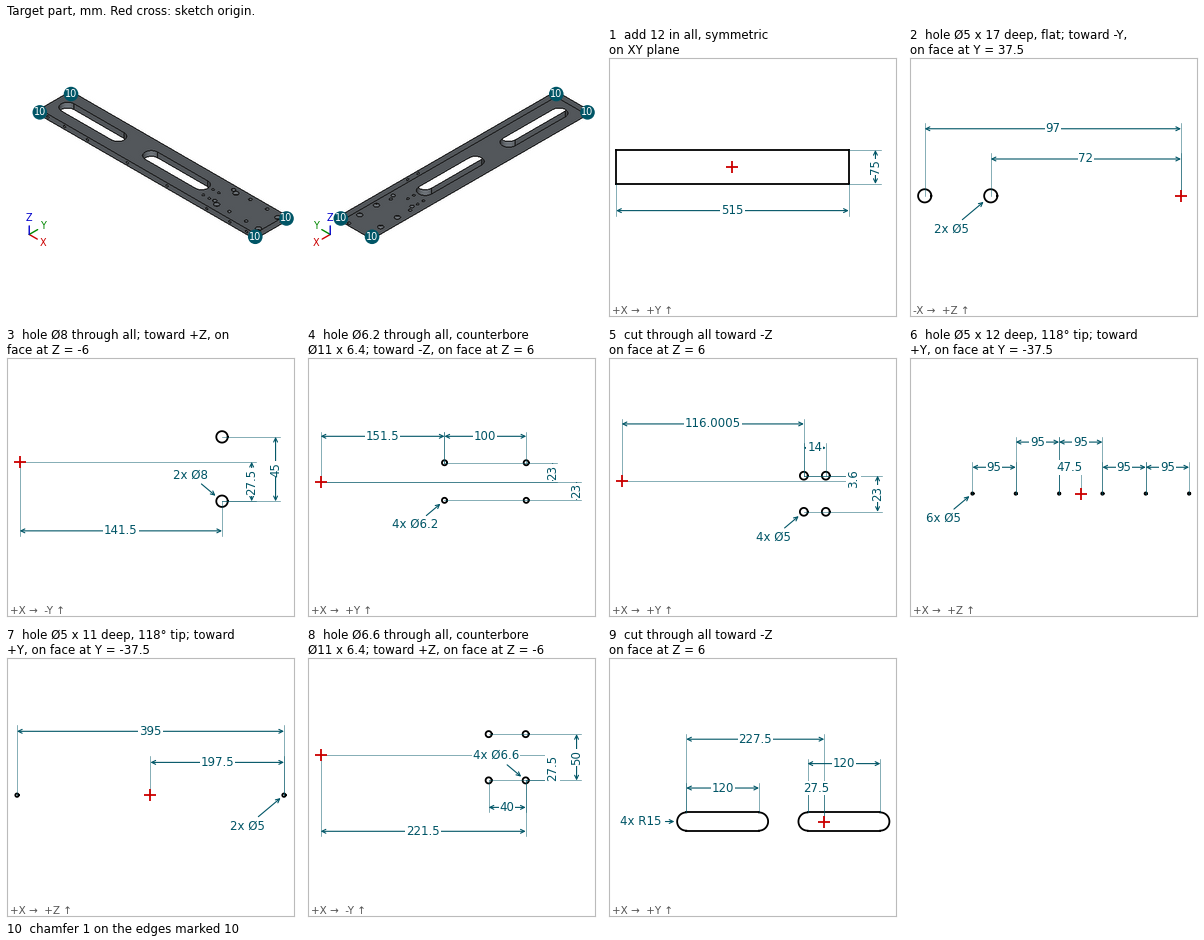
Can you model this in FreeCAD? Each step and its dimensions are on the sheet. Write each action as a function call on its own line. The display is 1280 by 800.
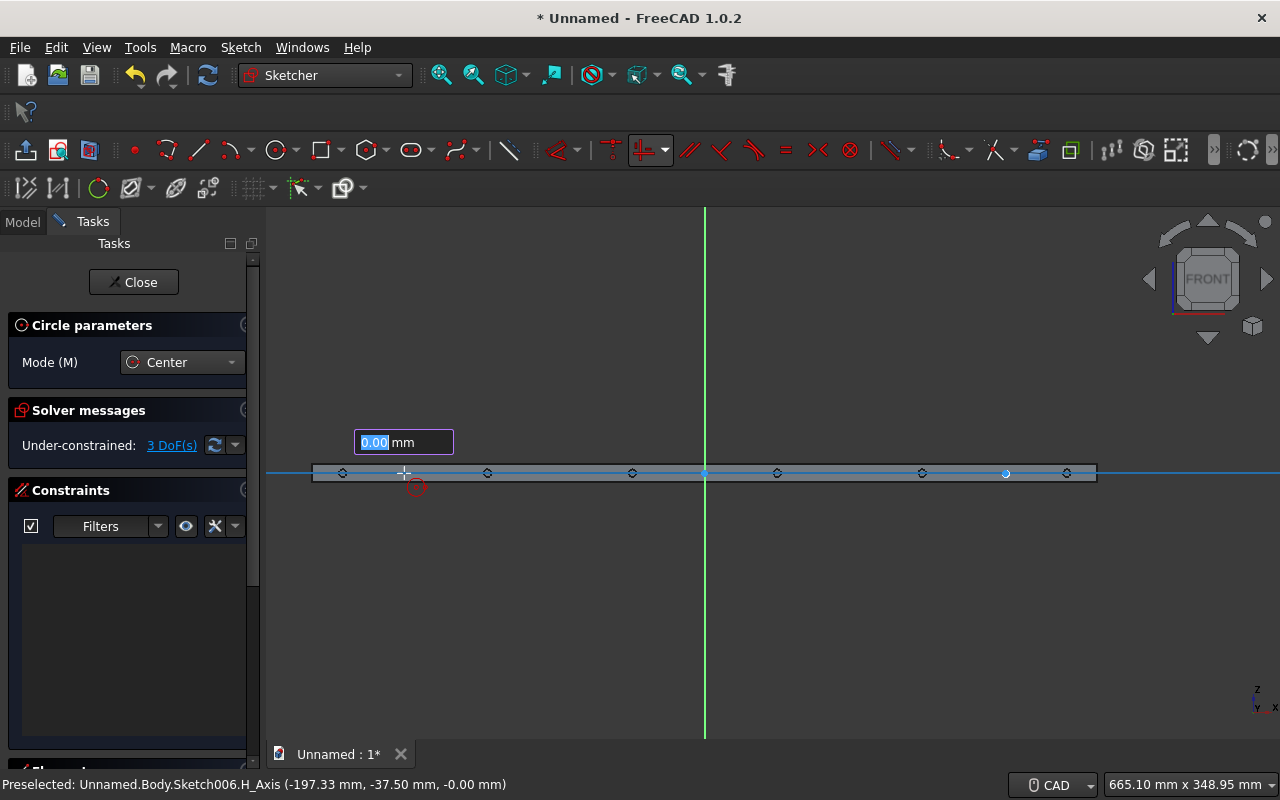
scroll(402, 477, up, 8)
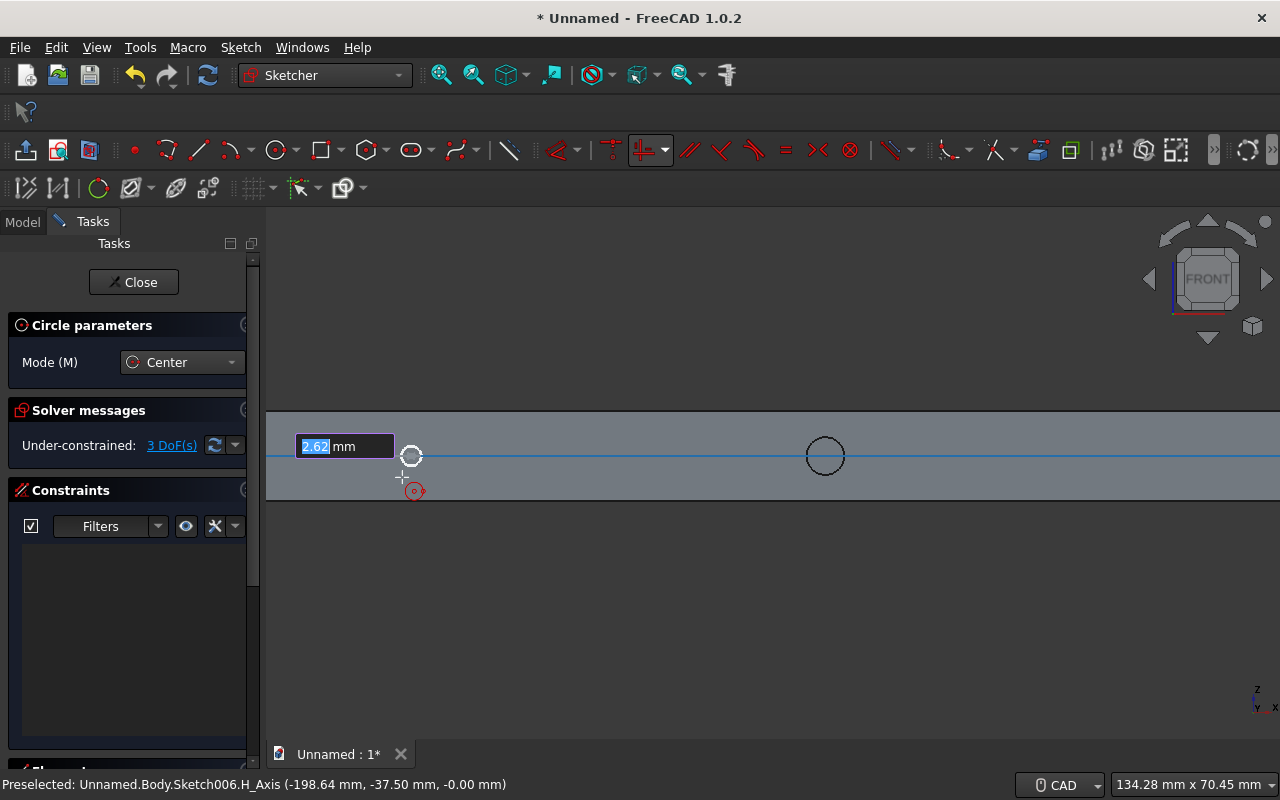
click(404, 474)
key(Escape)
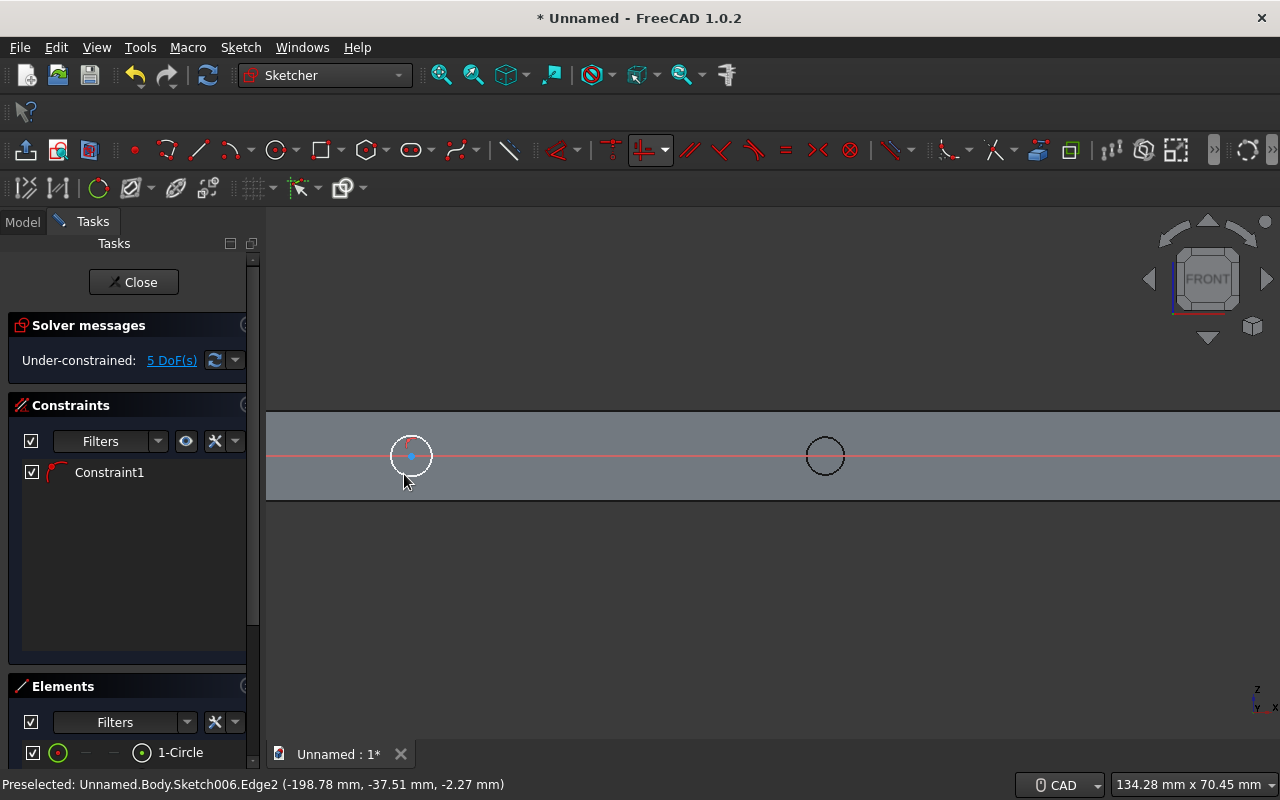
scroll(402, 477, down, 8)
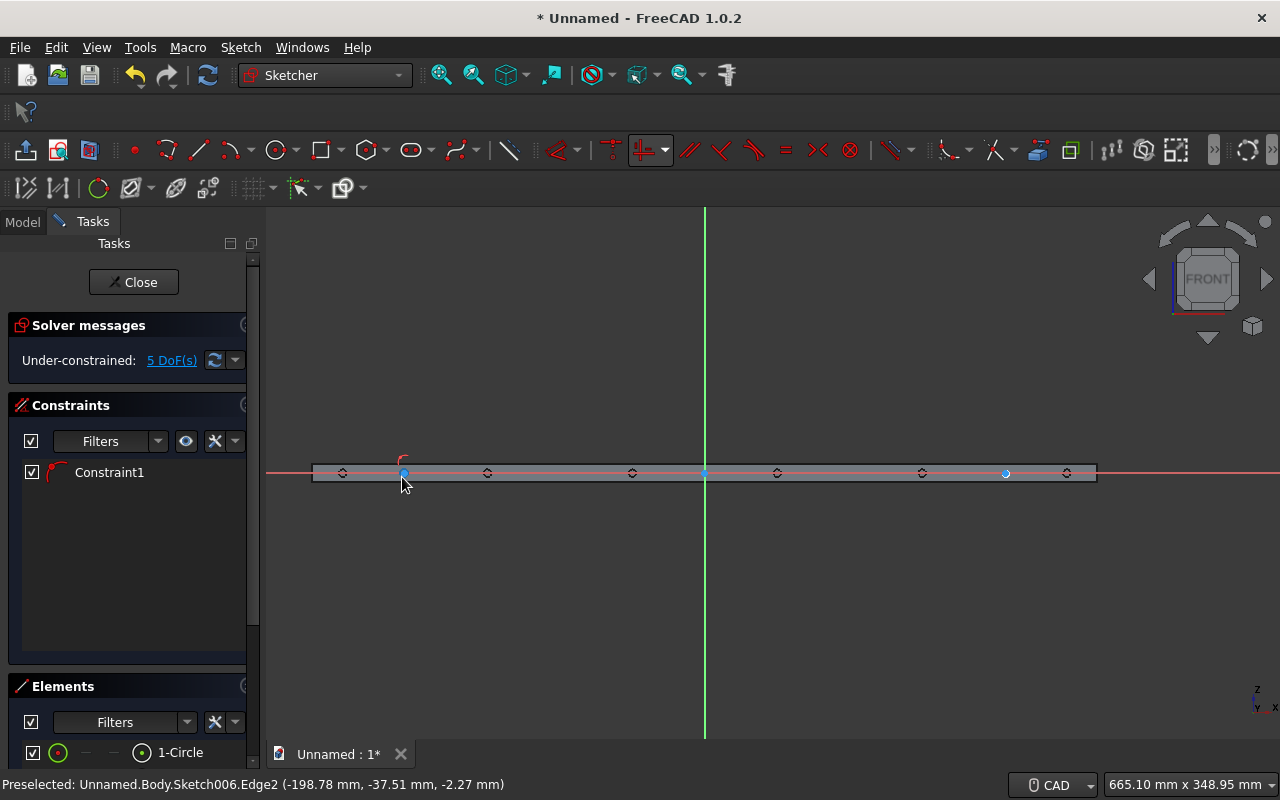
scroll(1004, 476, up, 8)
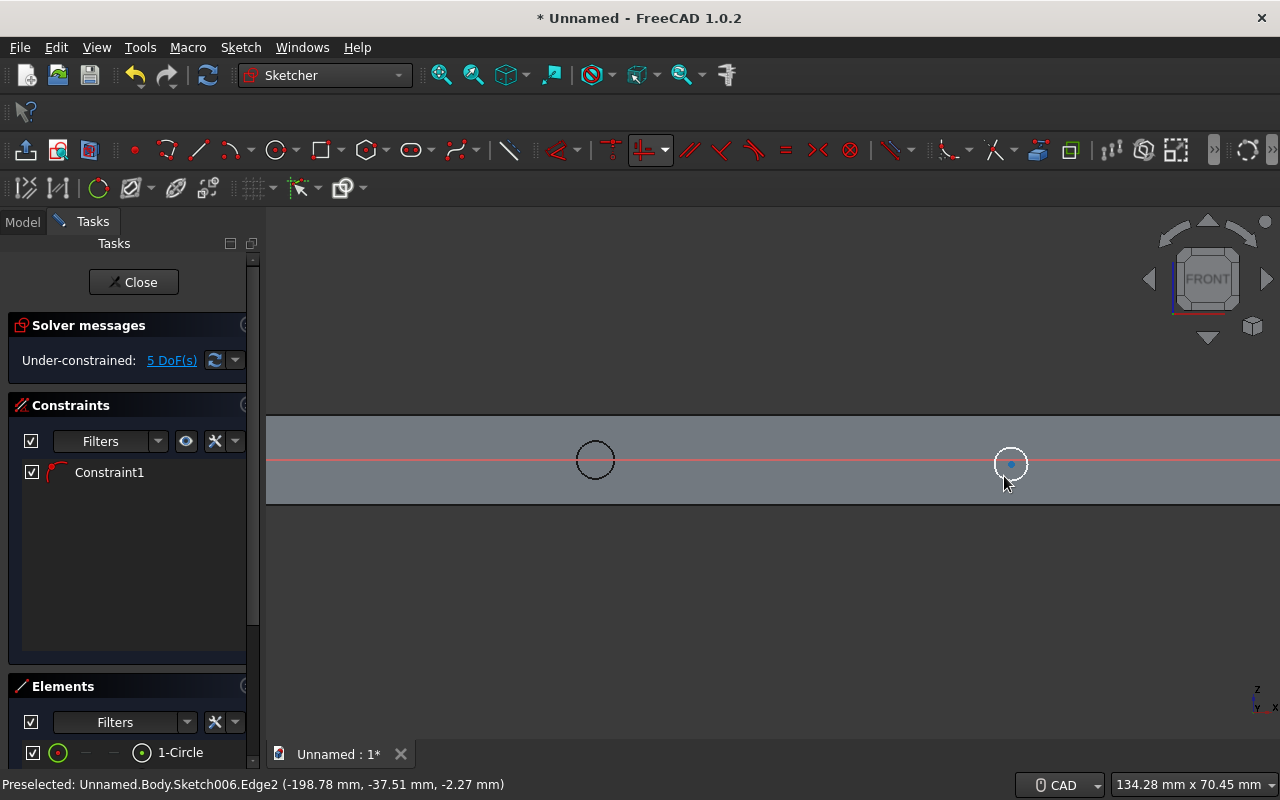
click(999, 476)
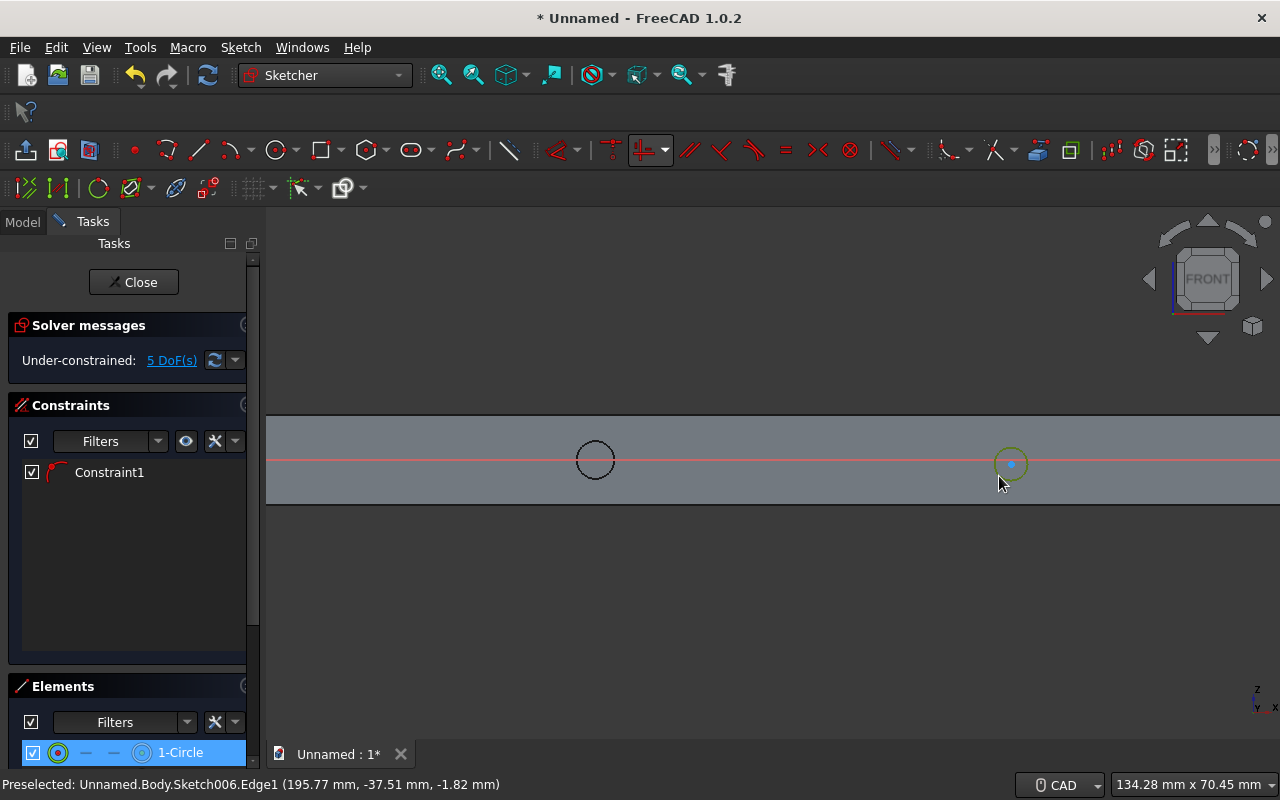
scroll(1004, 476, down, 8)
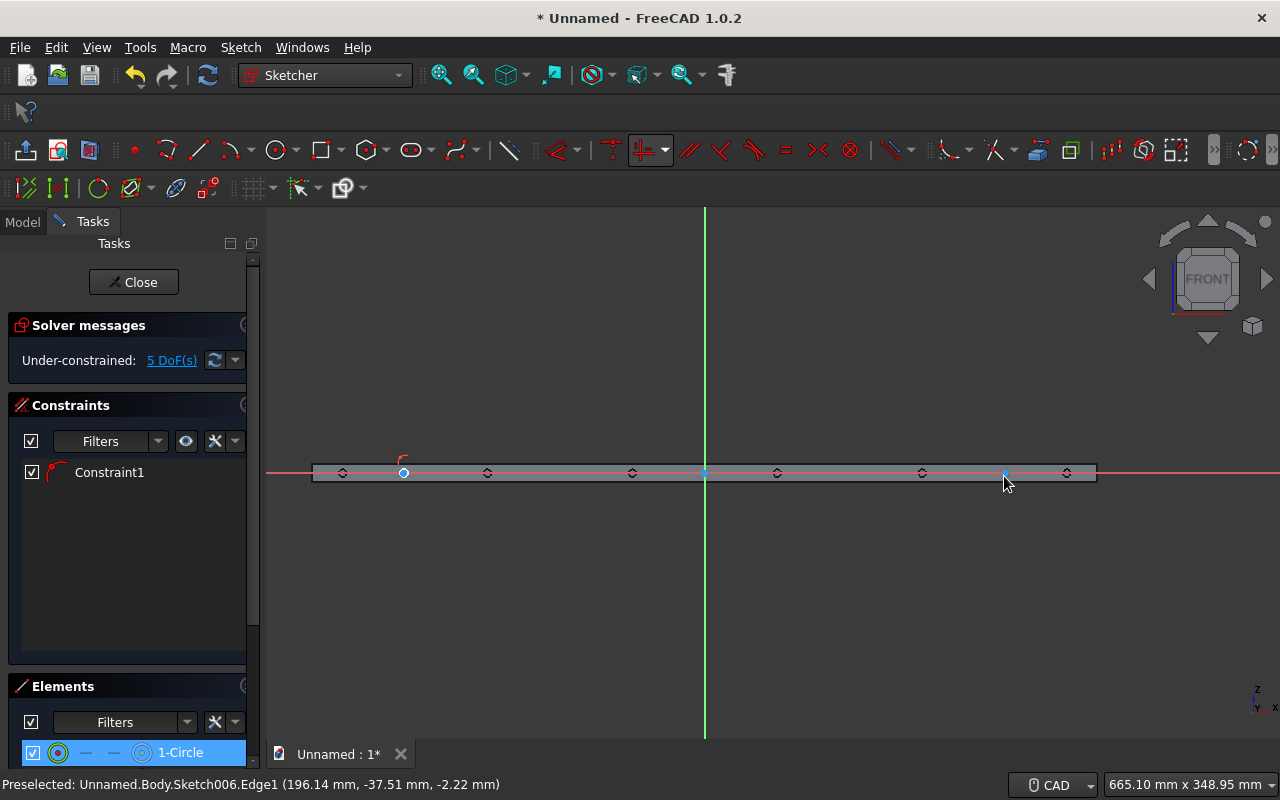
scroll(407, 470, up, 8)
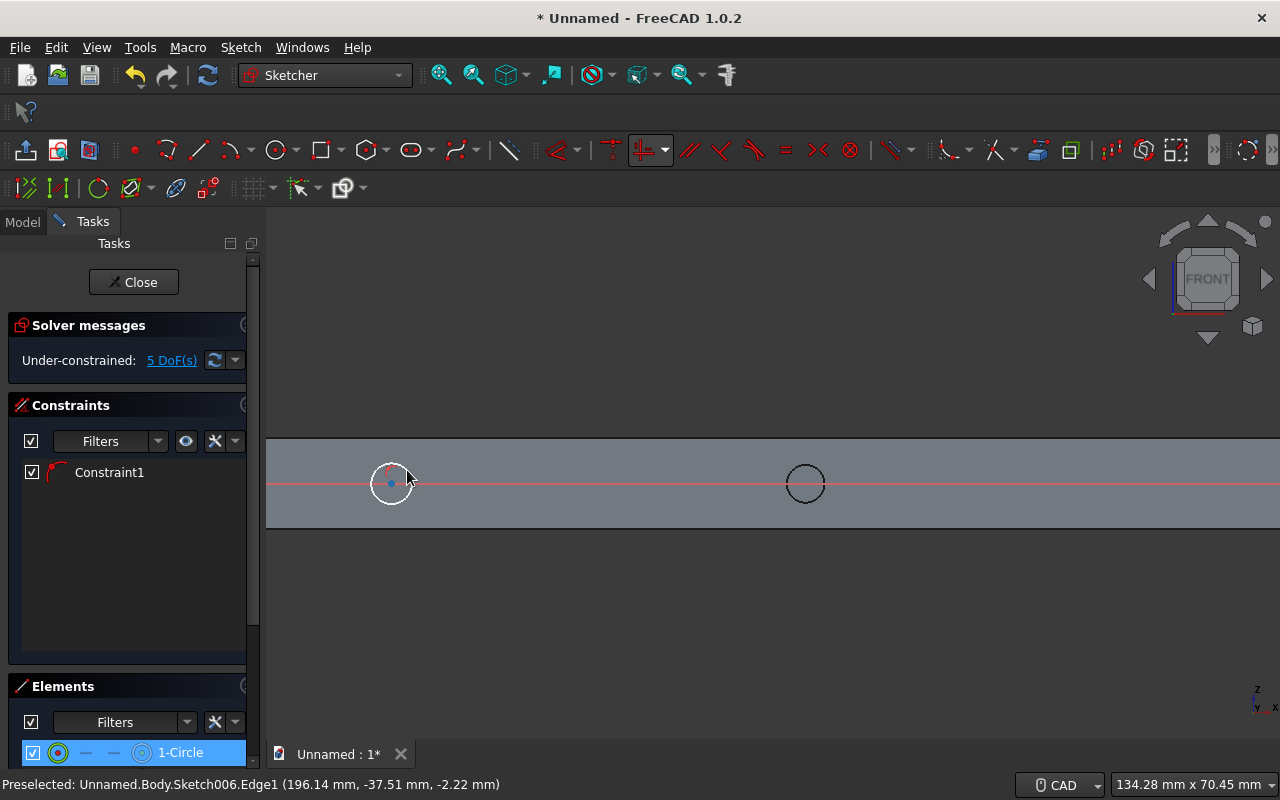
click(406, 469)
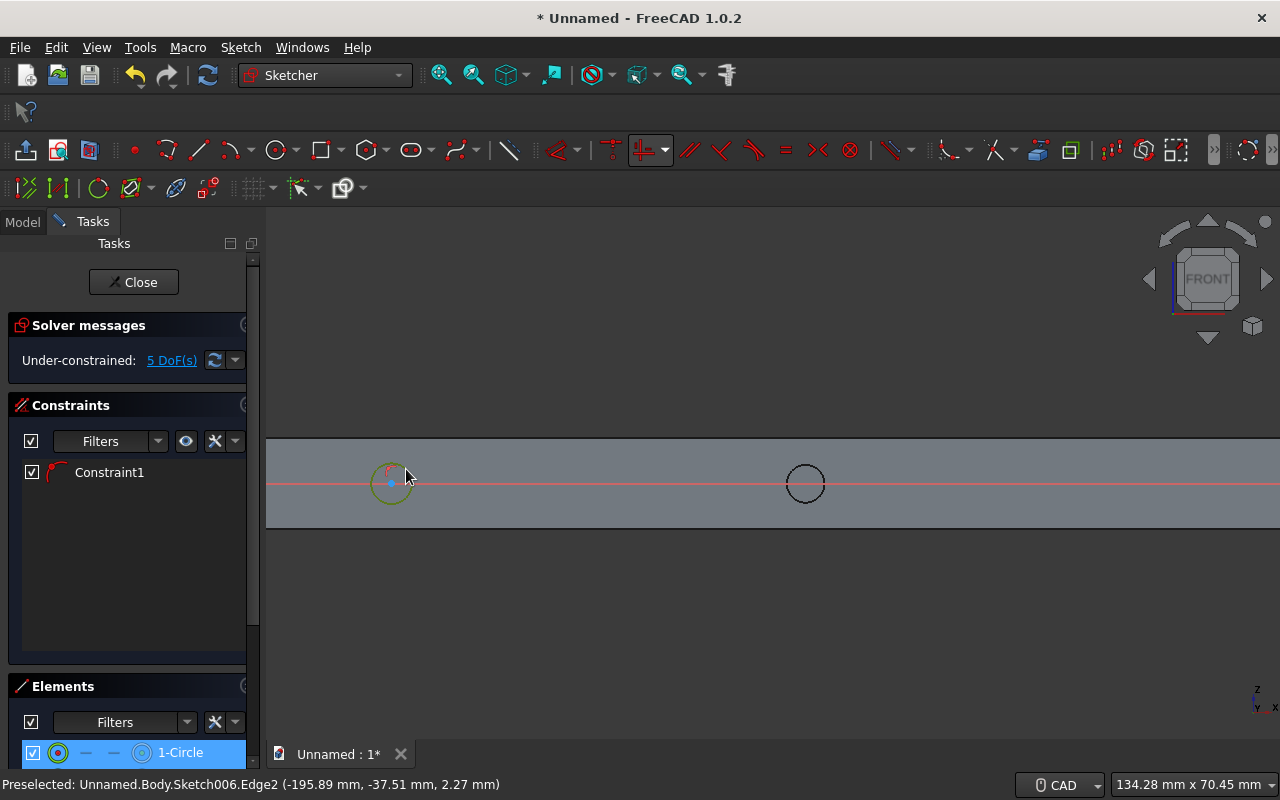
key(e)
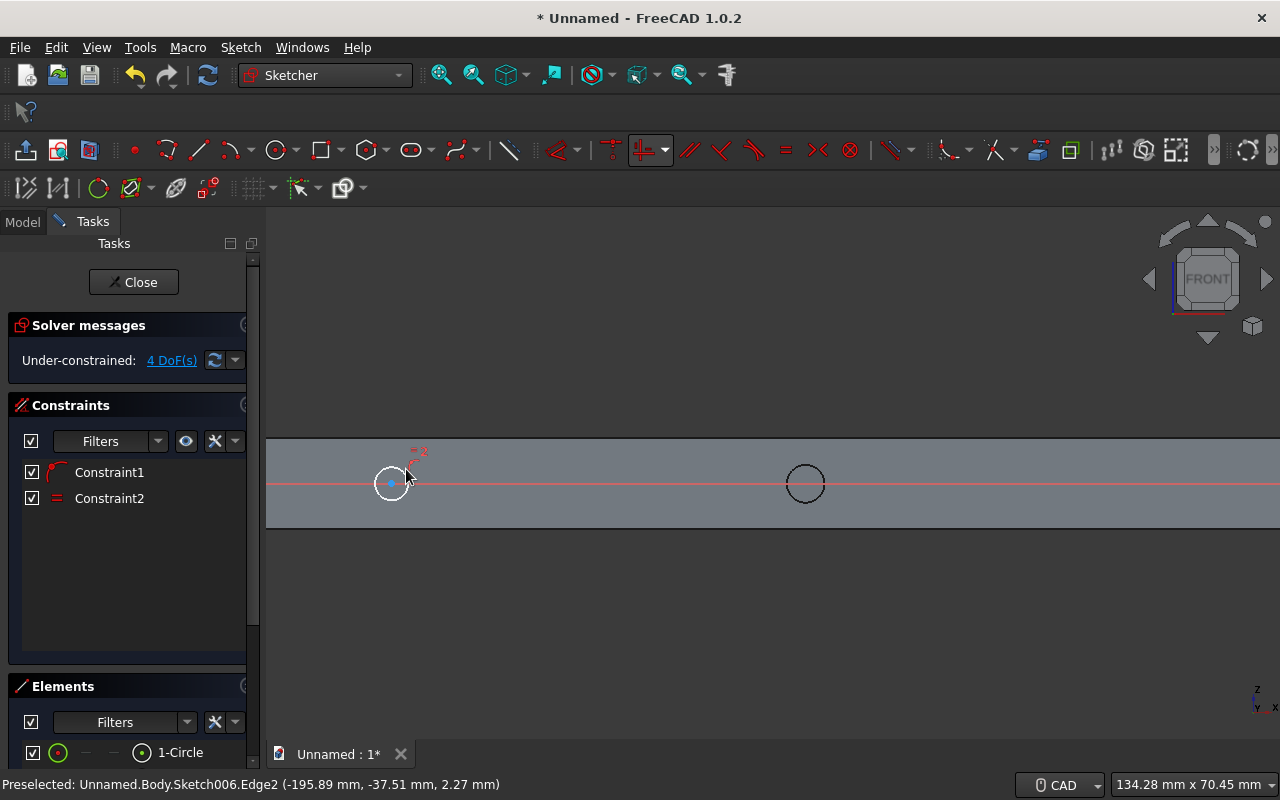
scroll(407, 470, down, 8)